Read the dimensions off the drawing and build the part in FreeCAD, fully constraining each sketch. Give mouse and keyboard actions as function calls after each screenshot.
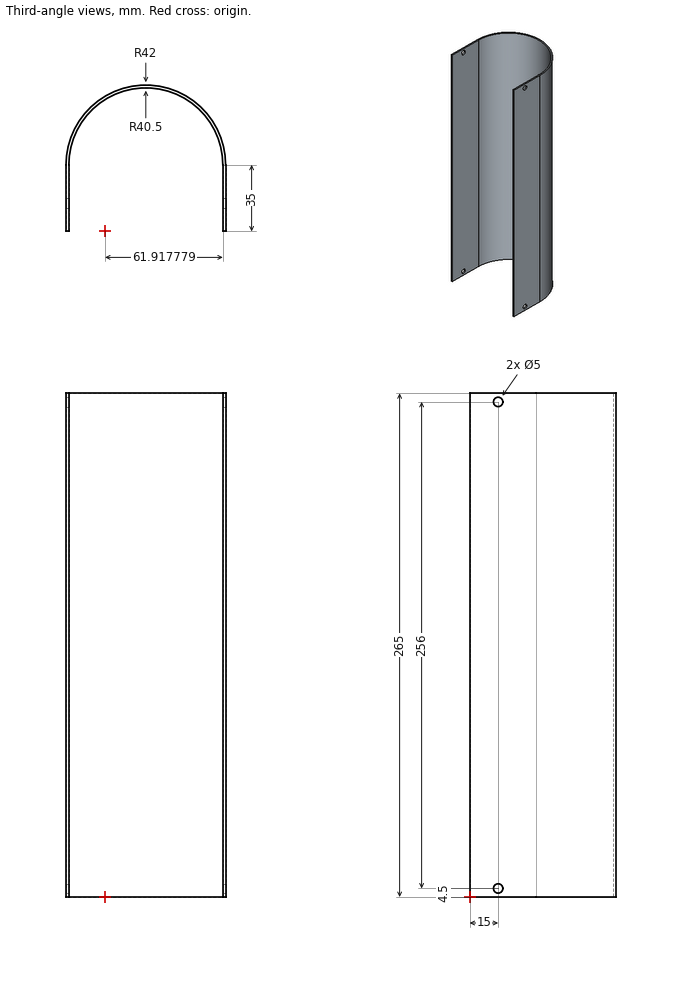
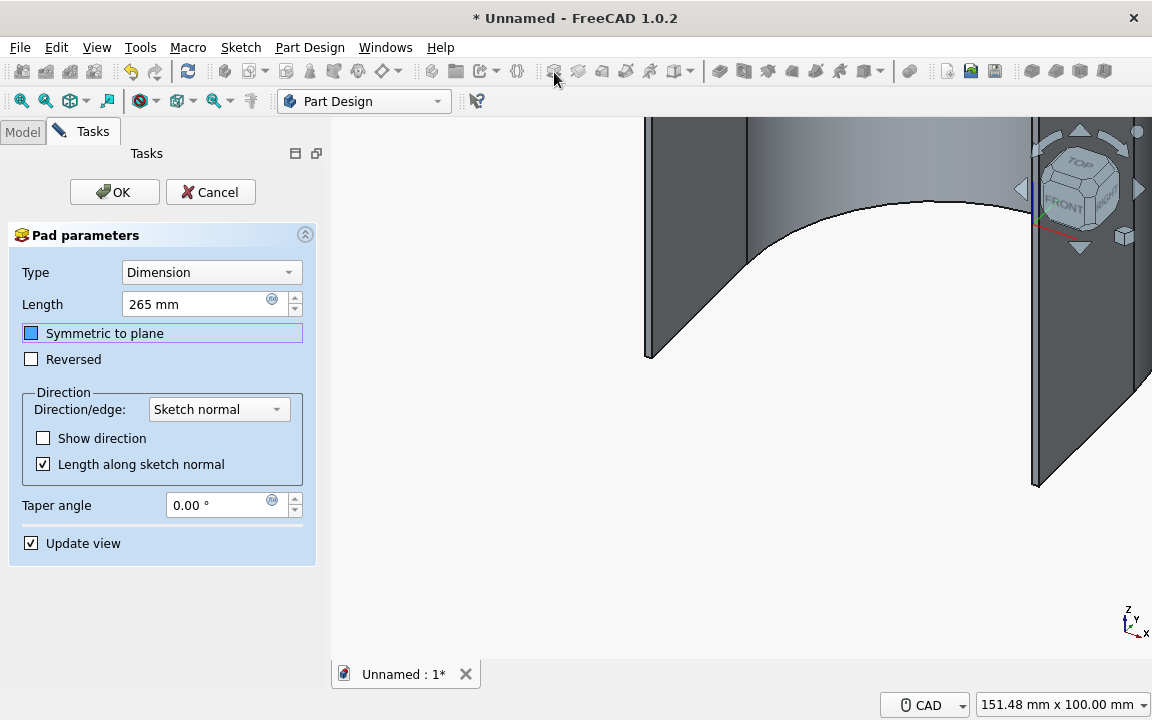
click(115, 192)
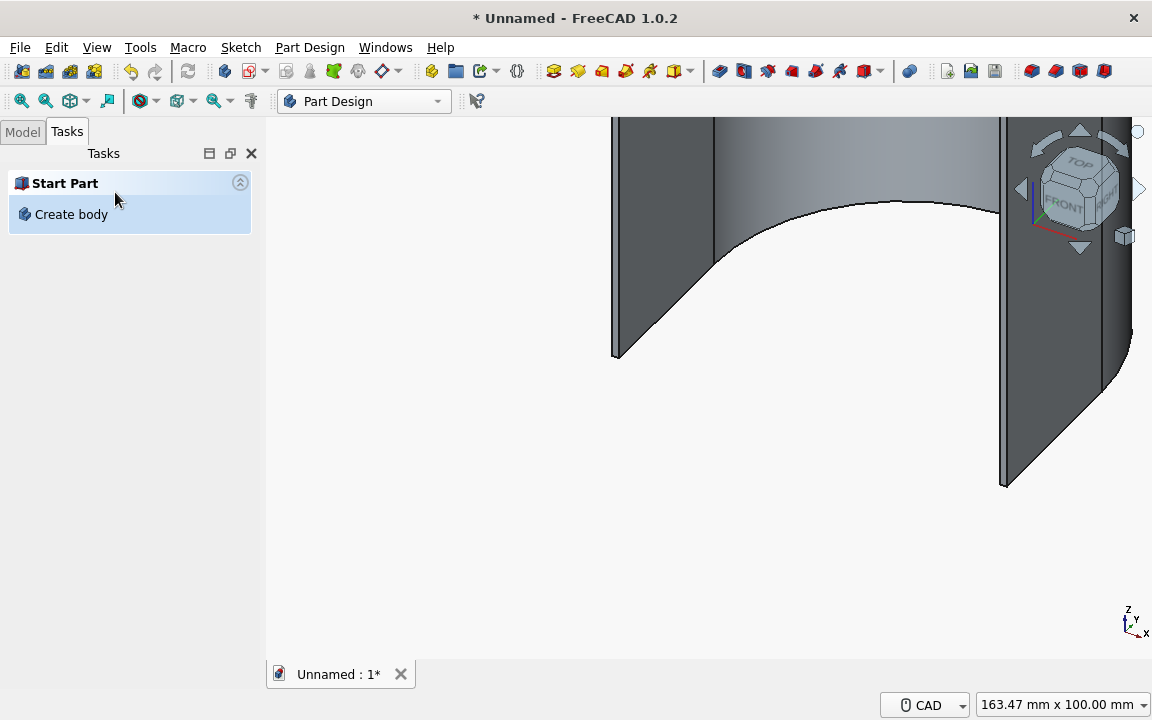
click(22, 102)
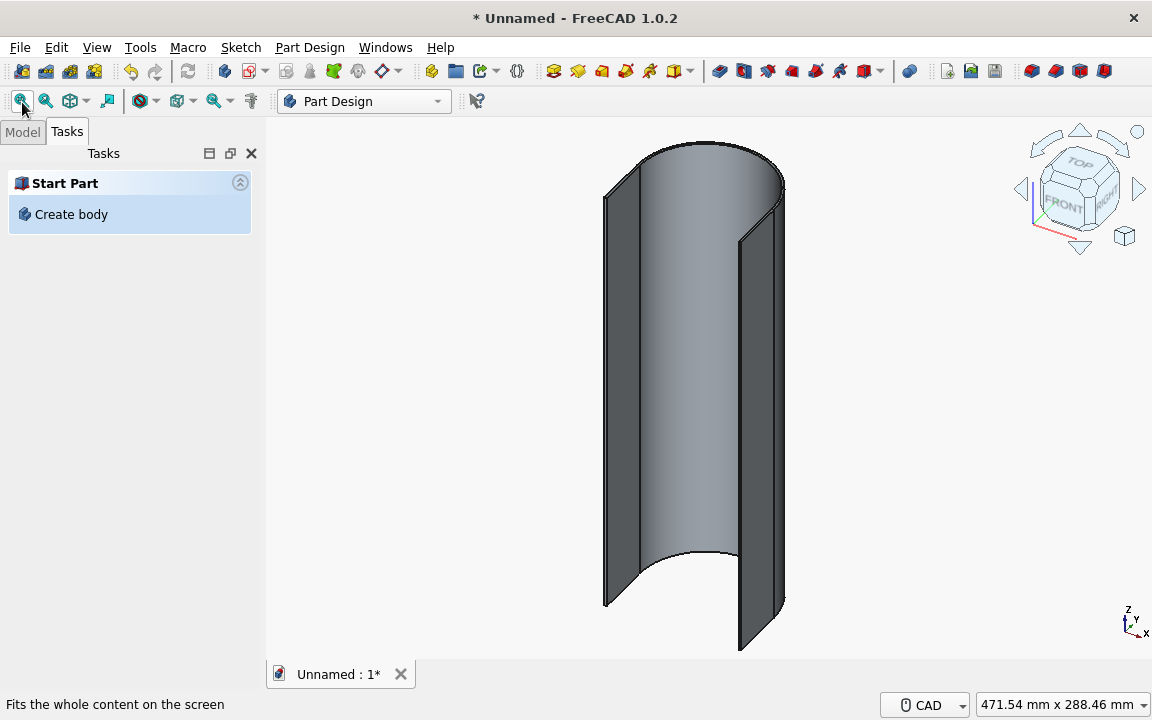
click(758, 254)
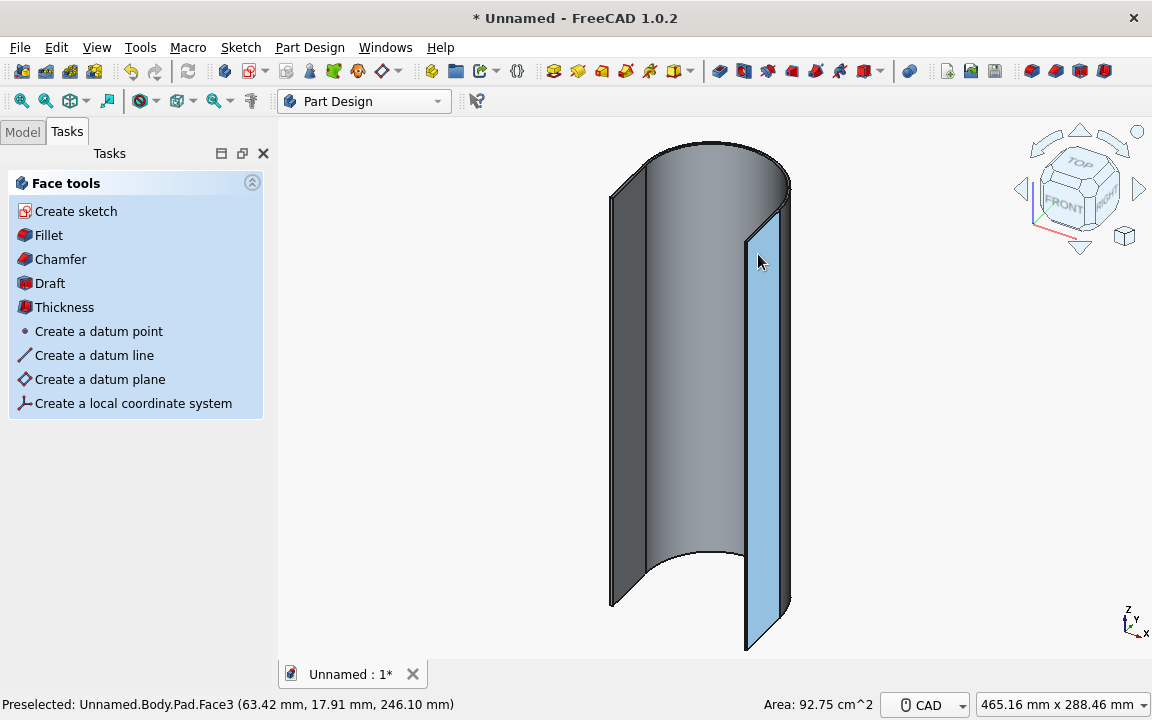
click(250, 72)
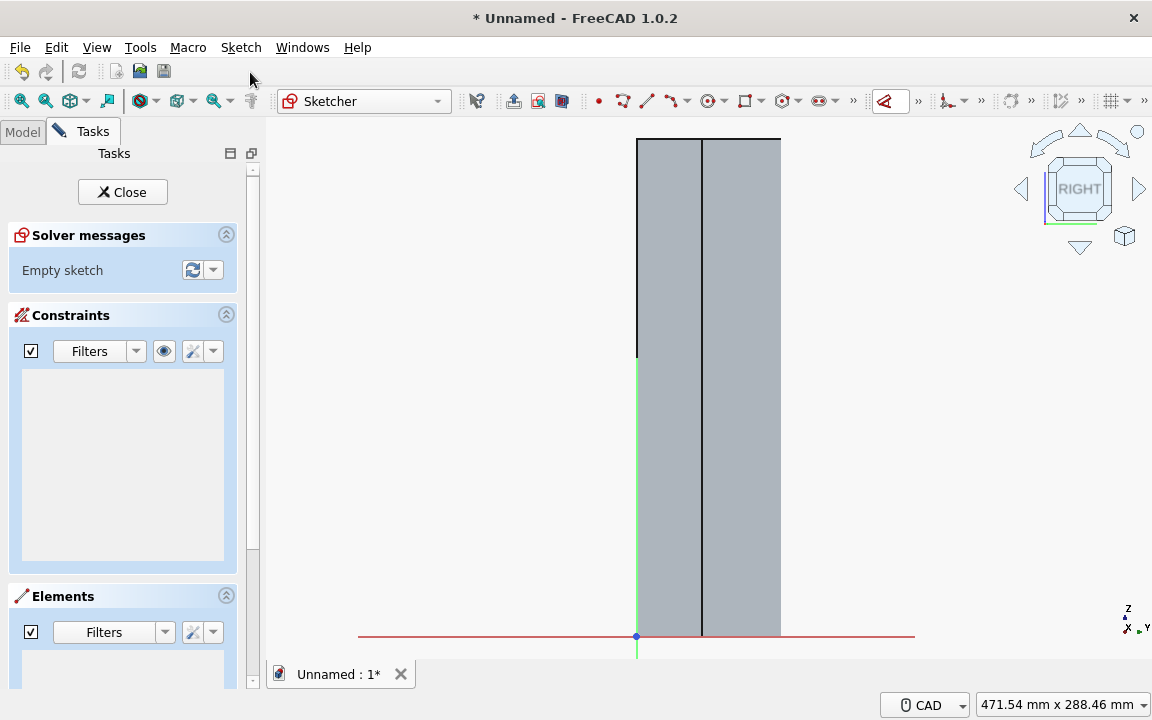
scroll(615, 384, down, 2)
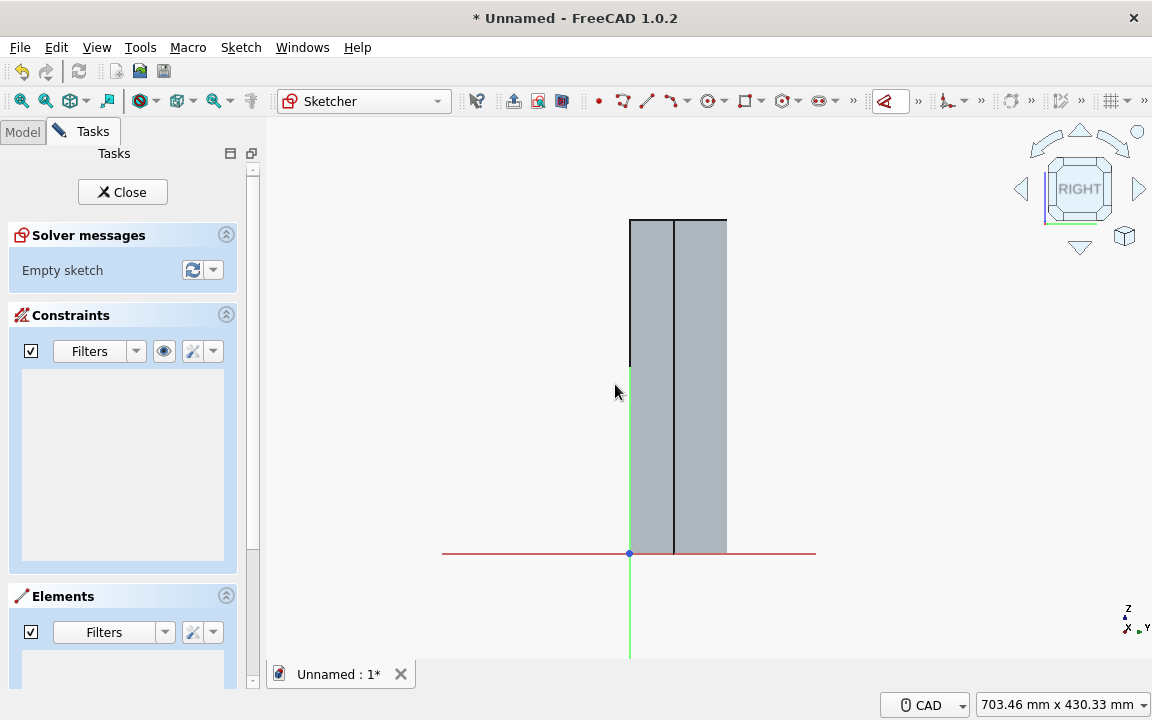
click(708, 102)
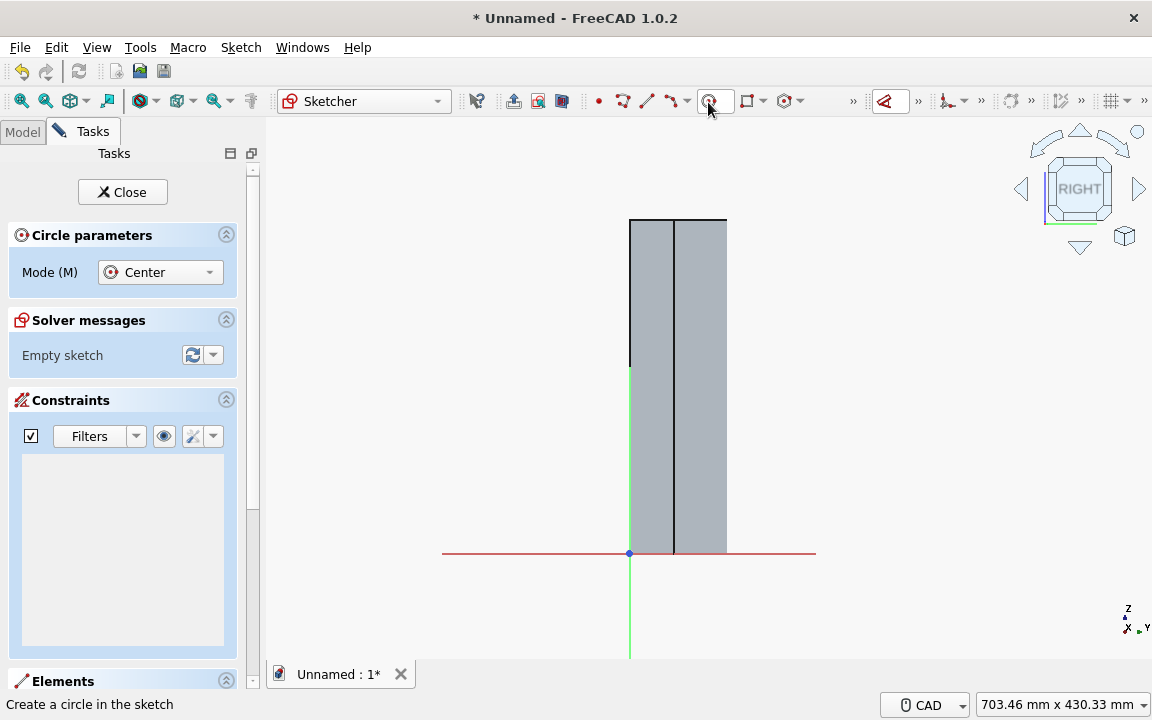
scroll(649, 226, up, 10)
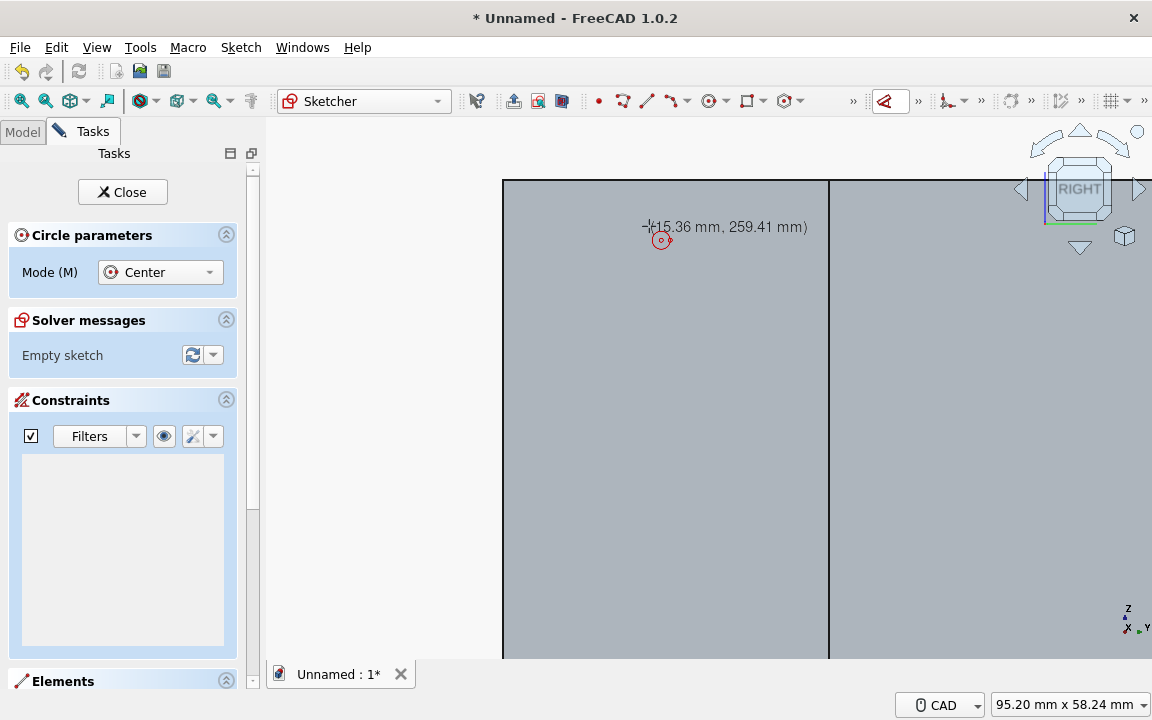
scroll(649, 226, down, 10)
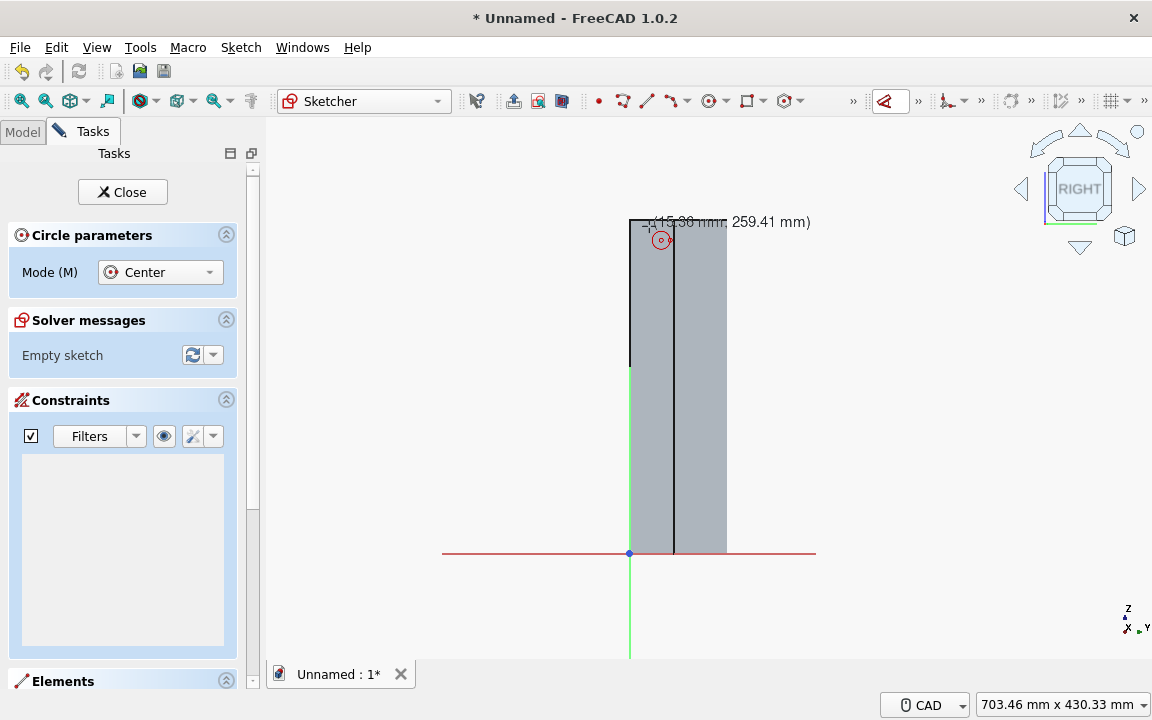
click(649, 226)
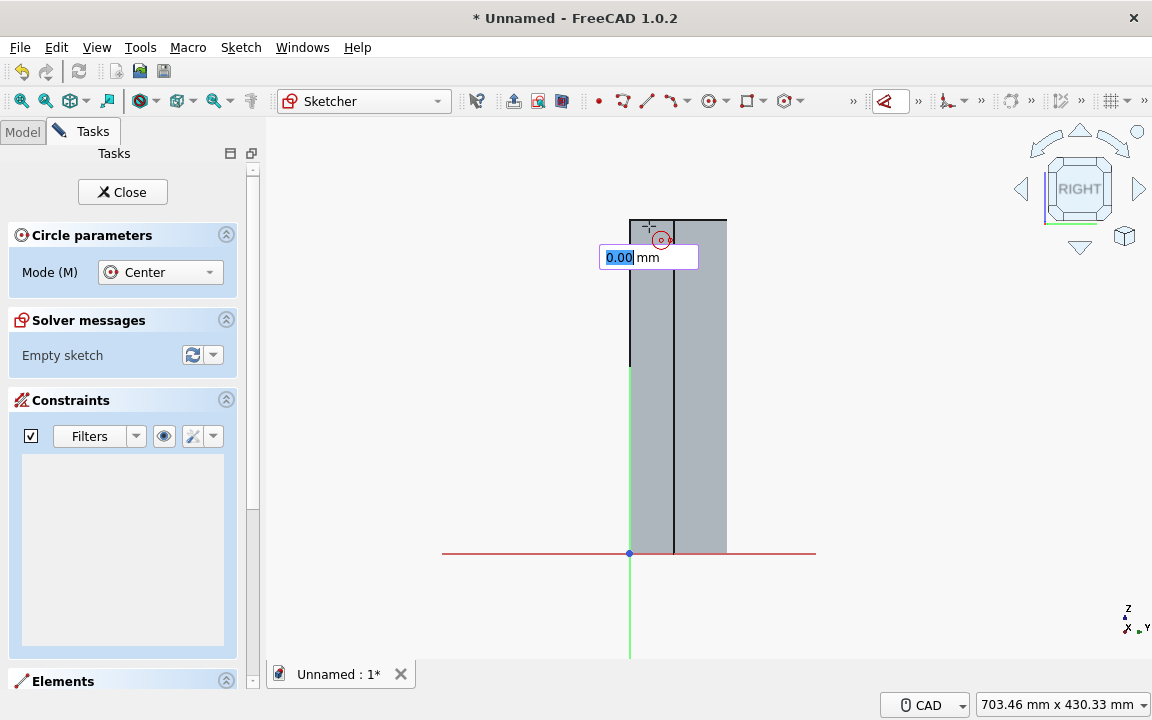
scroll(651, 223, up, 9)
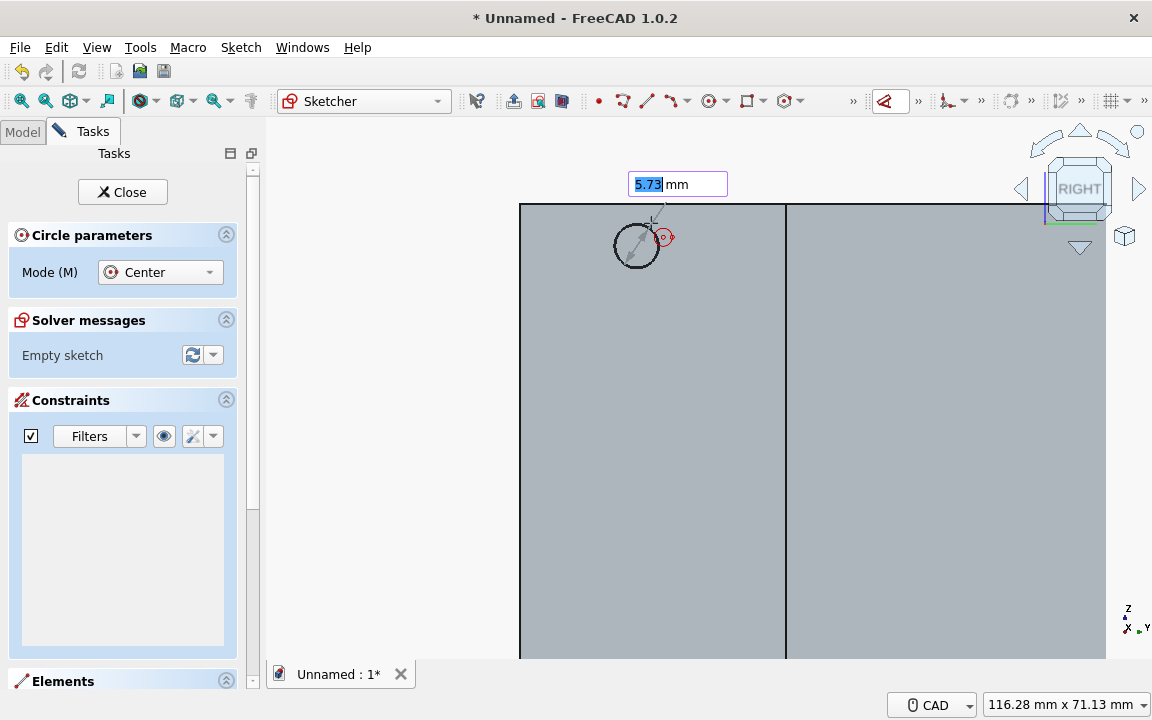
click(647, 224)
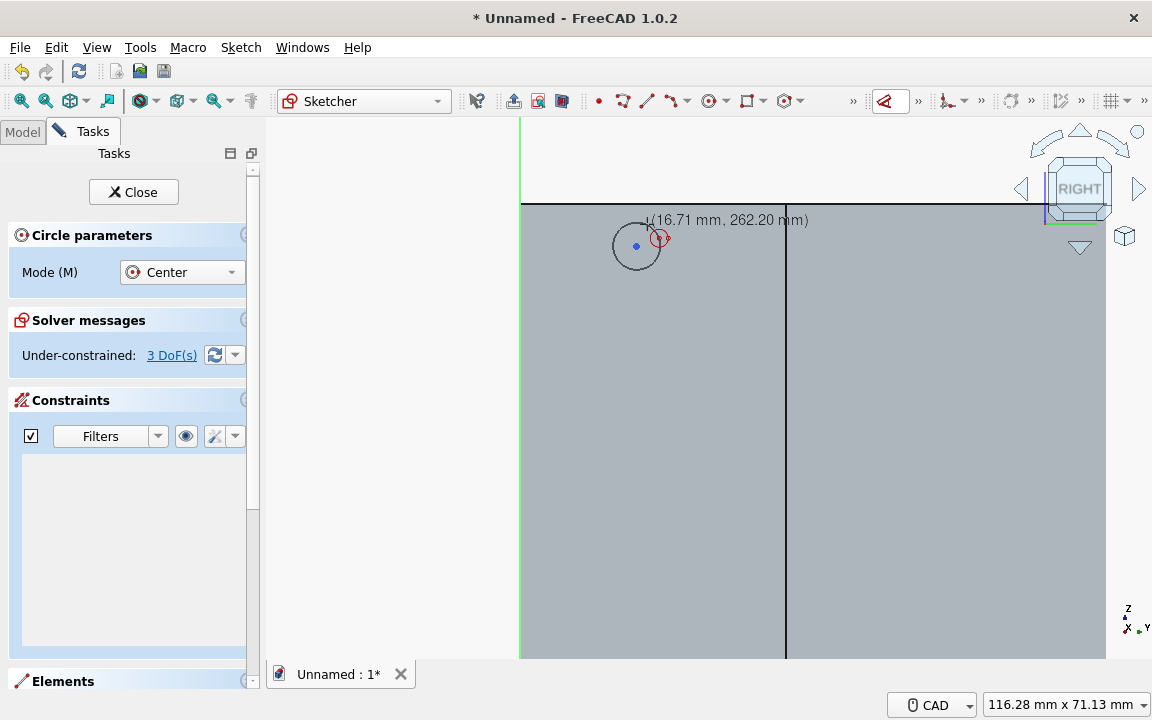
scroll(651, 223, down, 9)